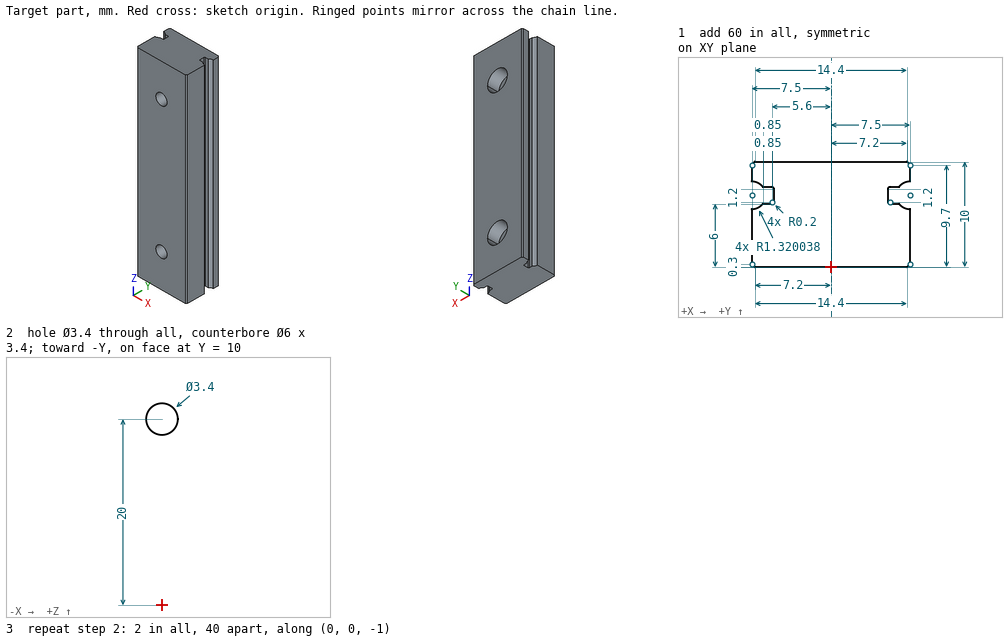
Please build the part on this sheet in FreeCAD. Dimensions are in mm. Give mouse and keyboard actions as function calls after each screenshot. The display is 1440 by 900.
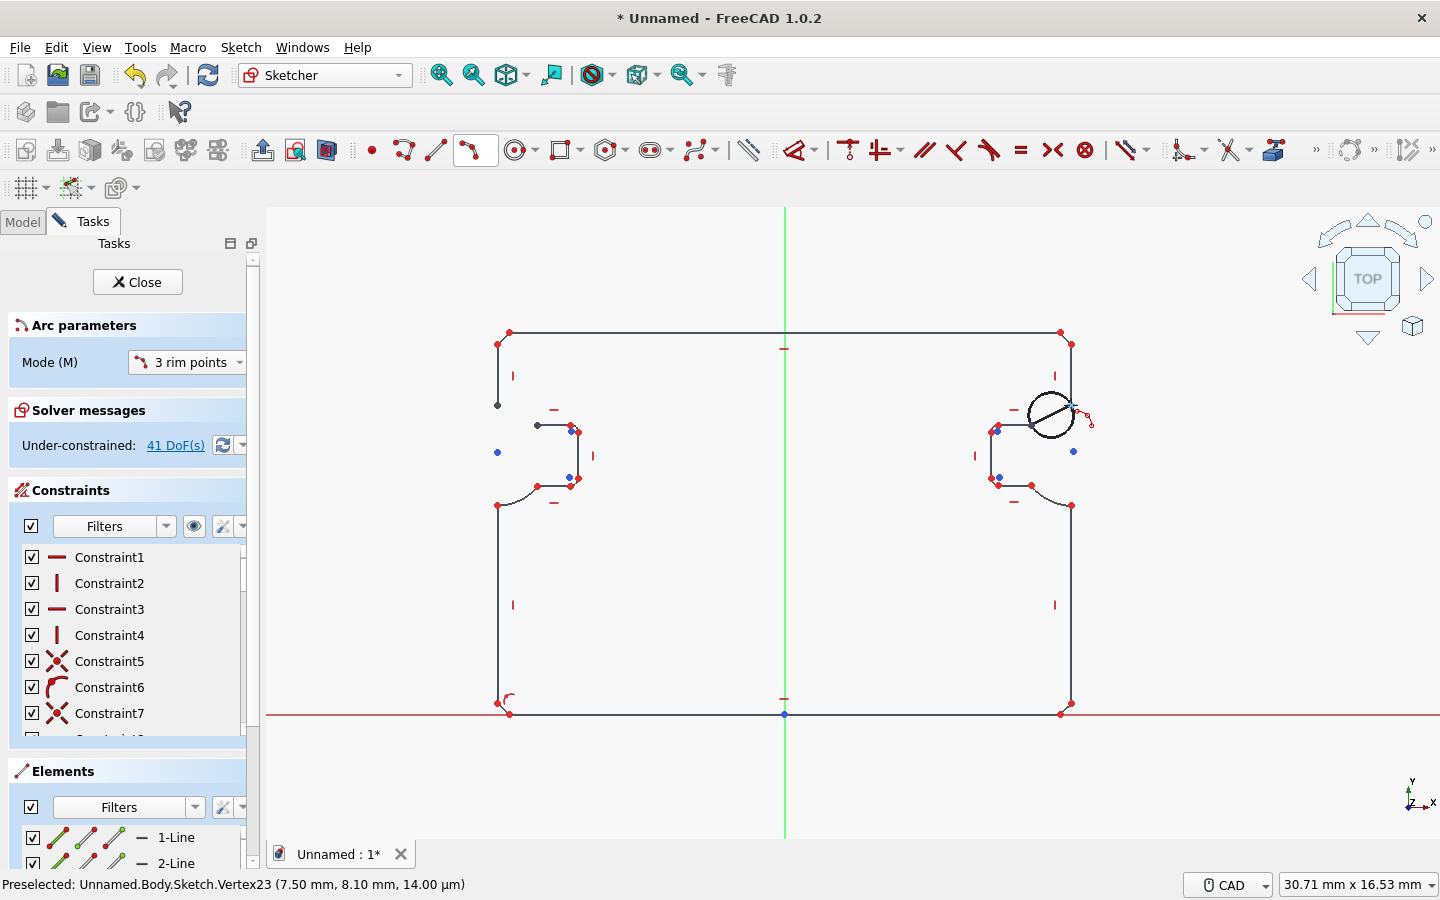
scroll(1049, 410, up, 6)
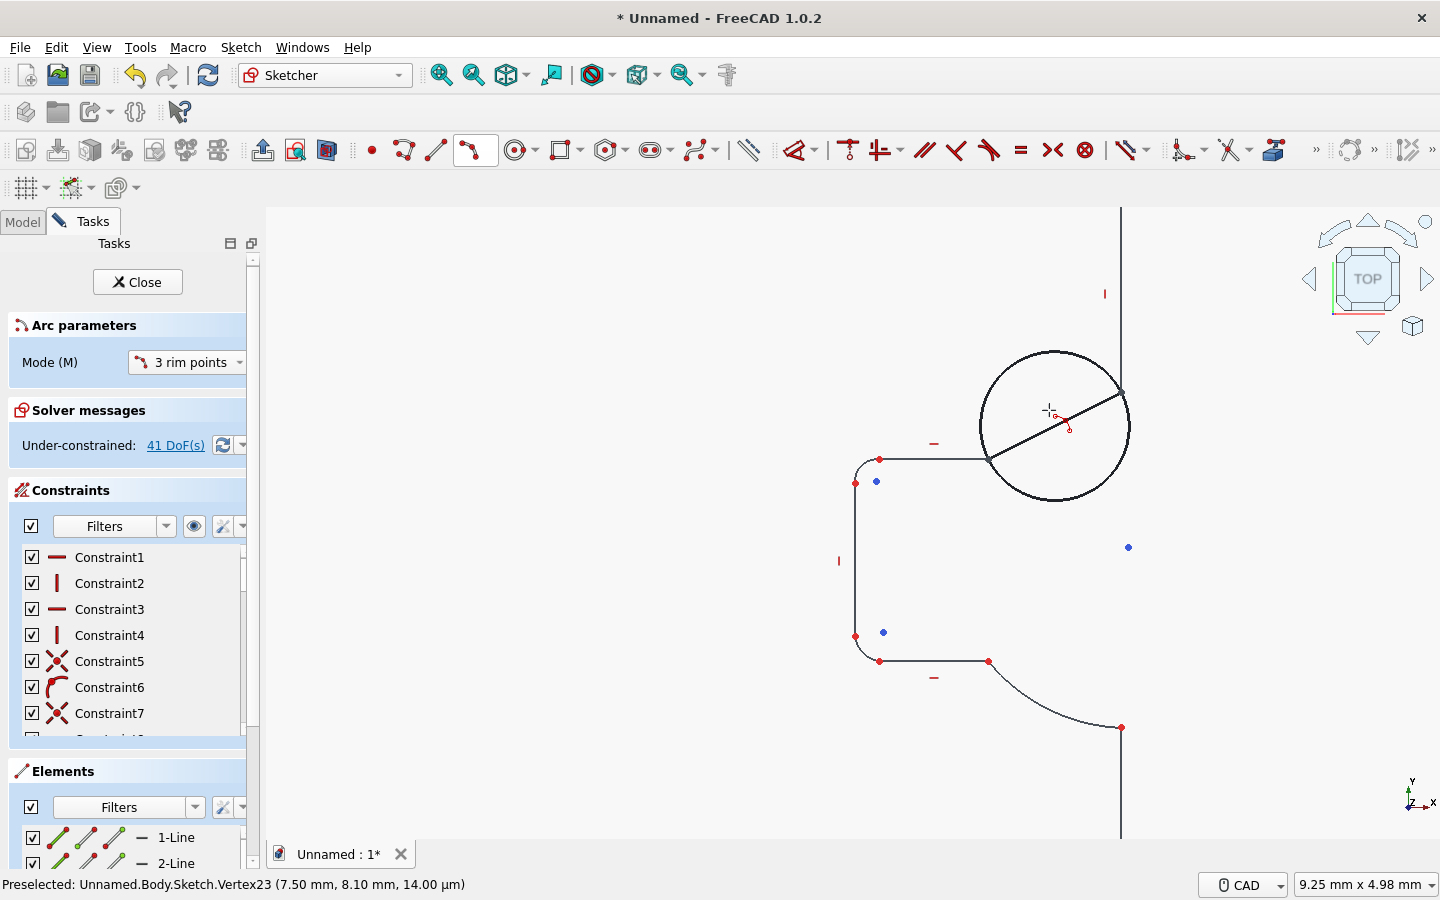
click(1047, 408)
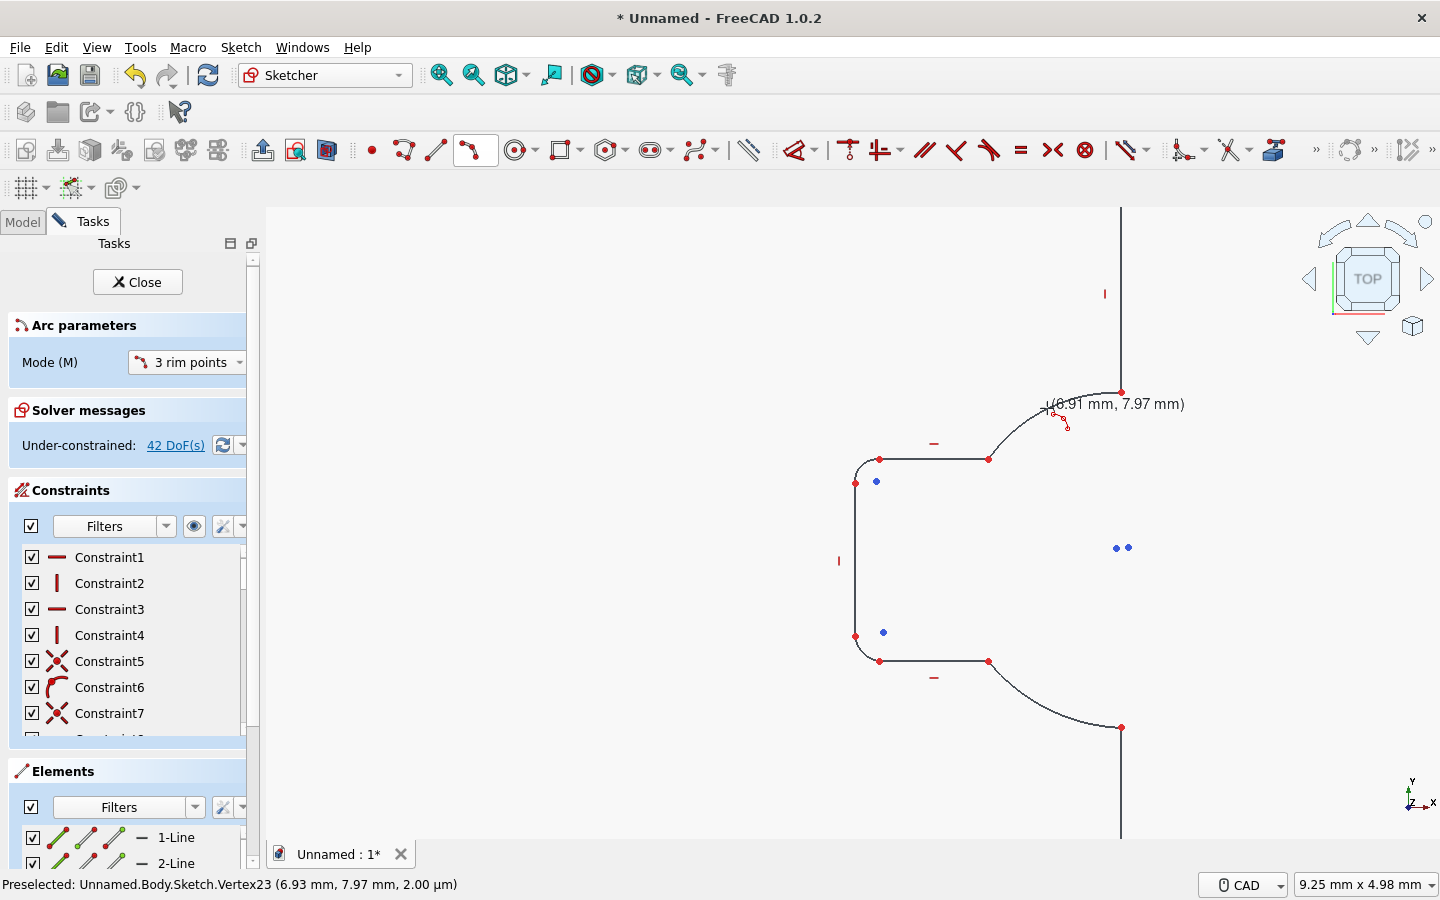
scroll(1049, 409, down, 6)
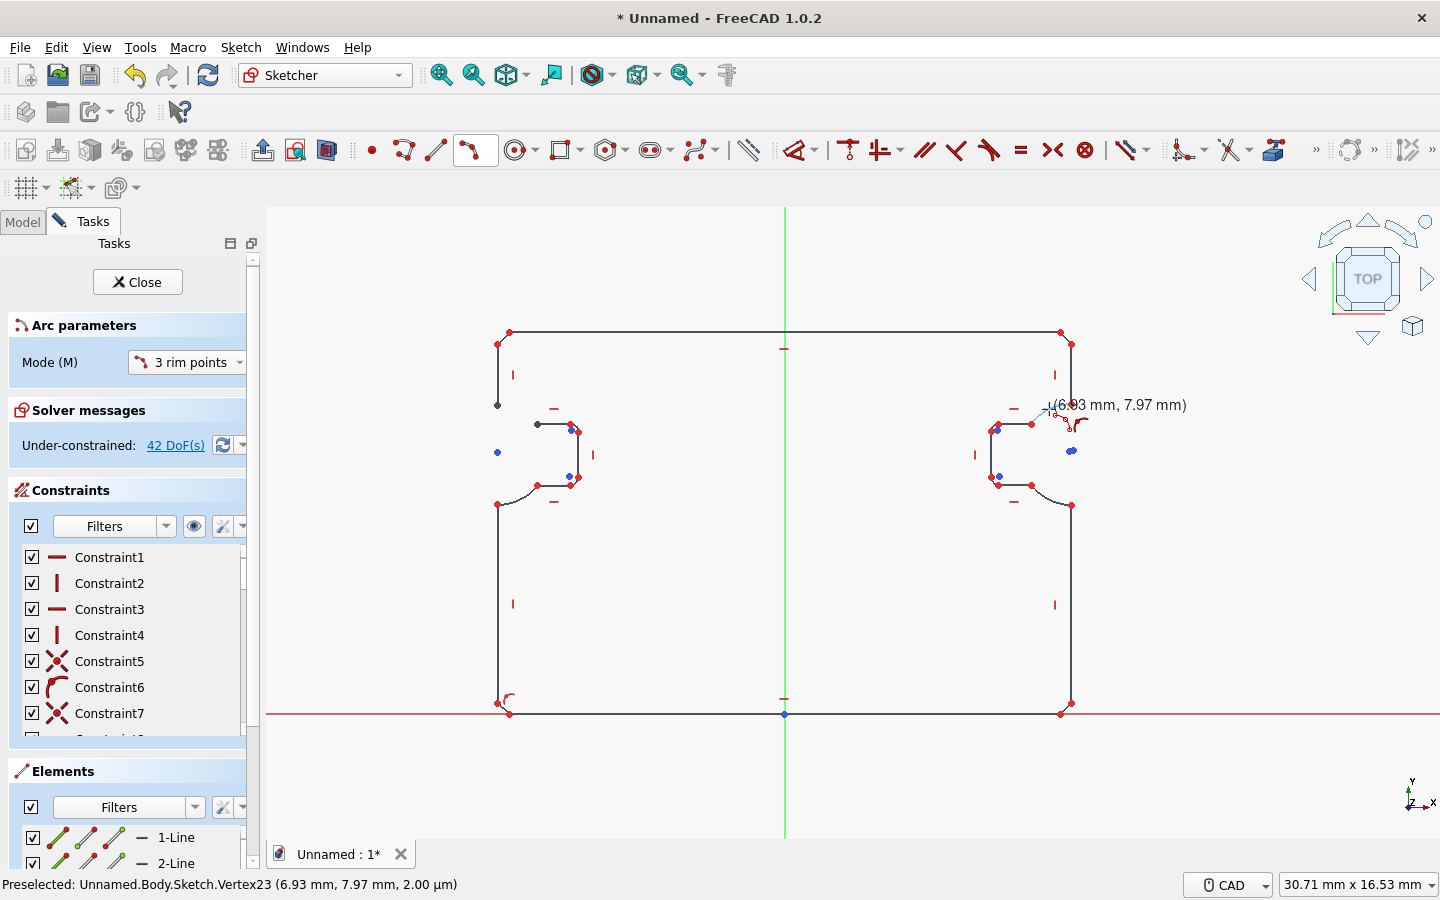
click(498, 405)
click(538, 424)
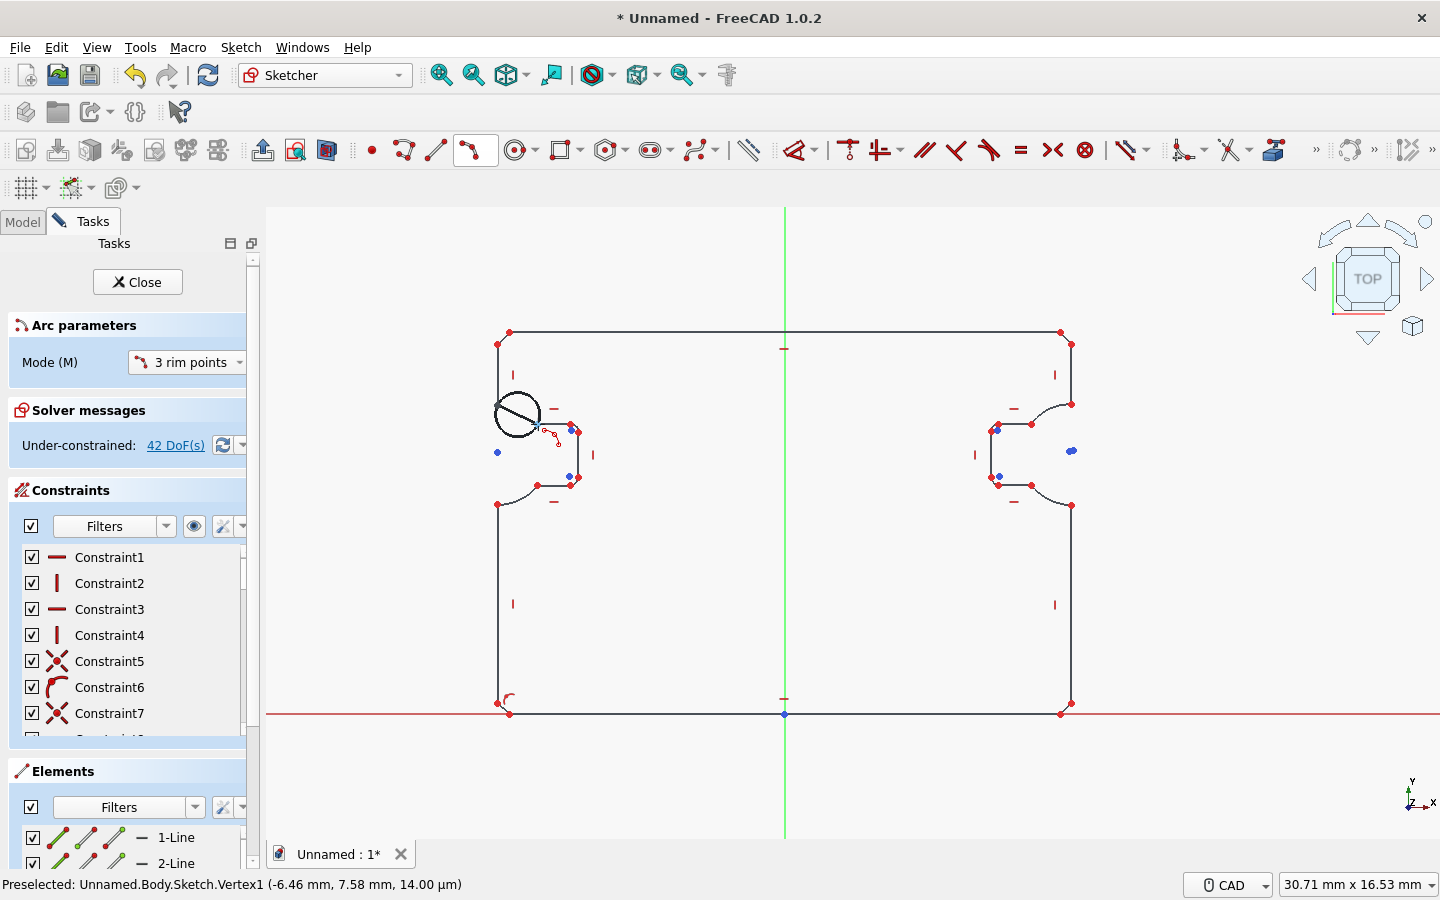
scroll(520, 409, up, 6)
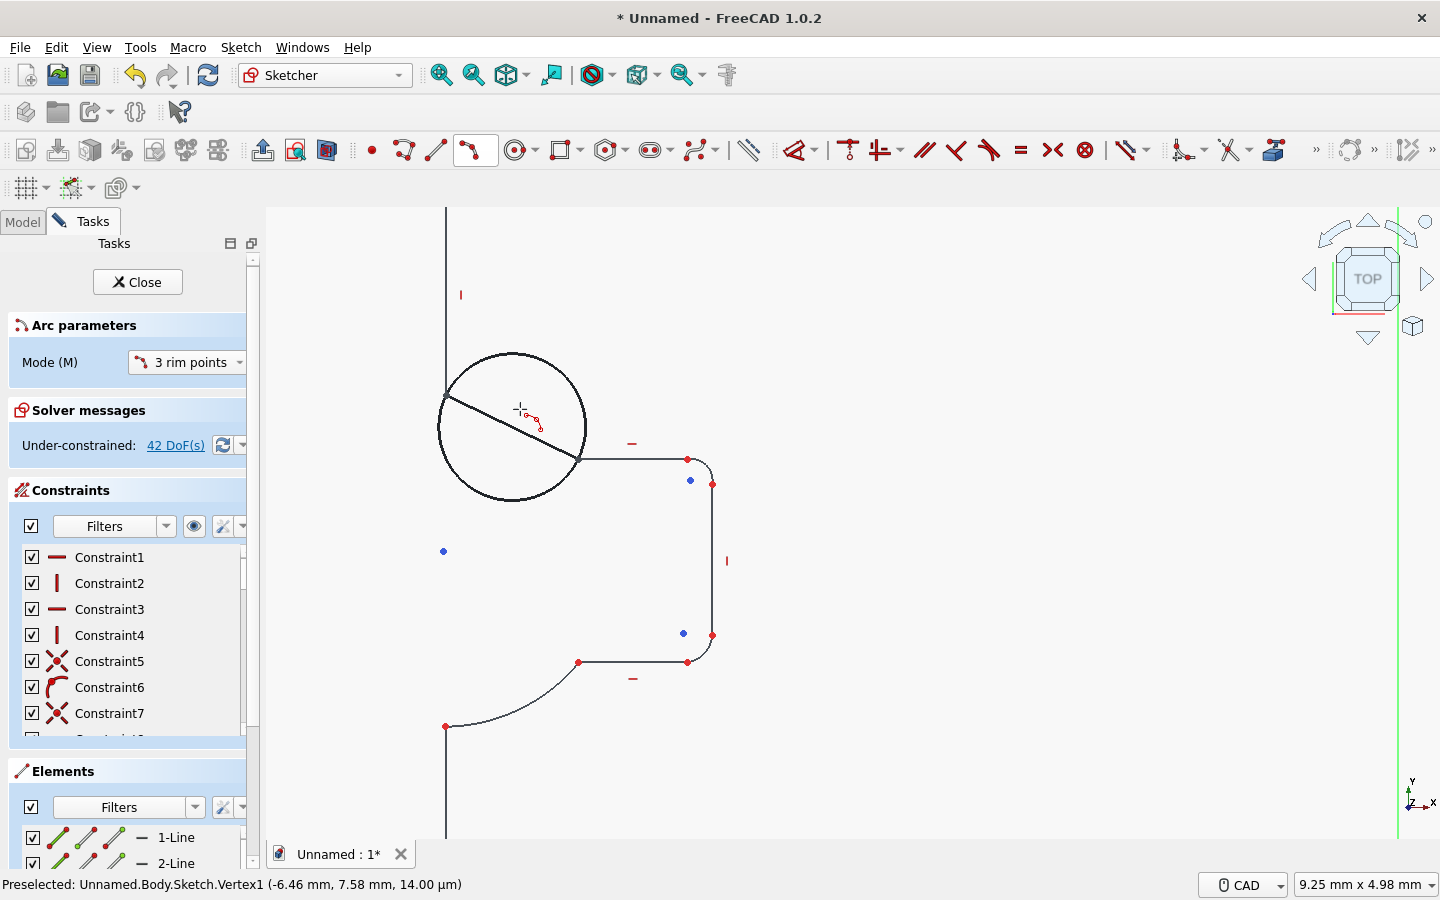
click(520, 408)
key(Escape)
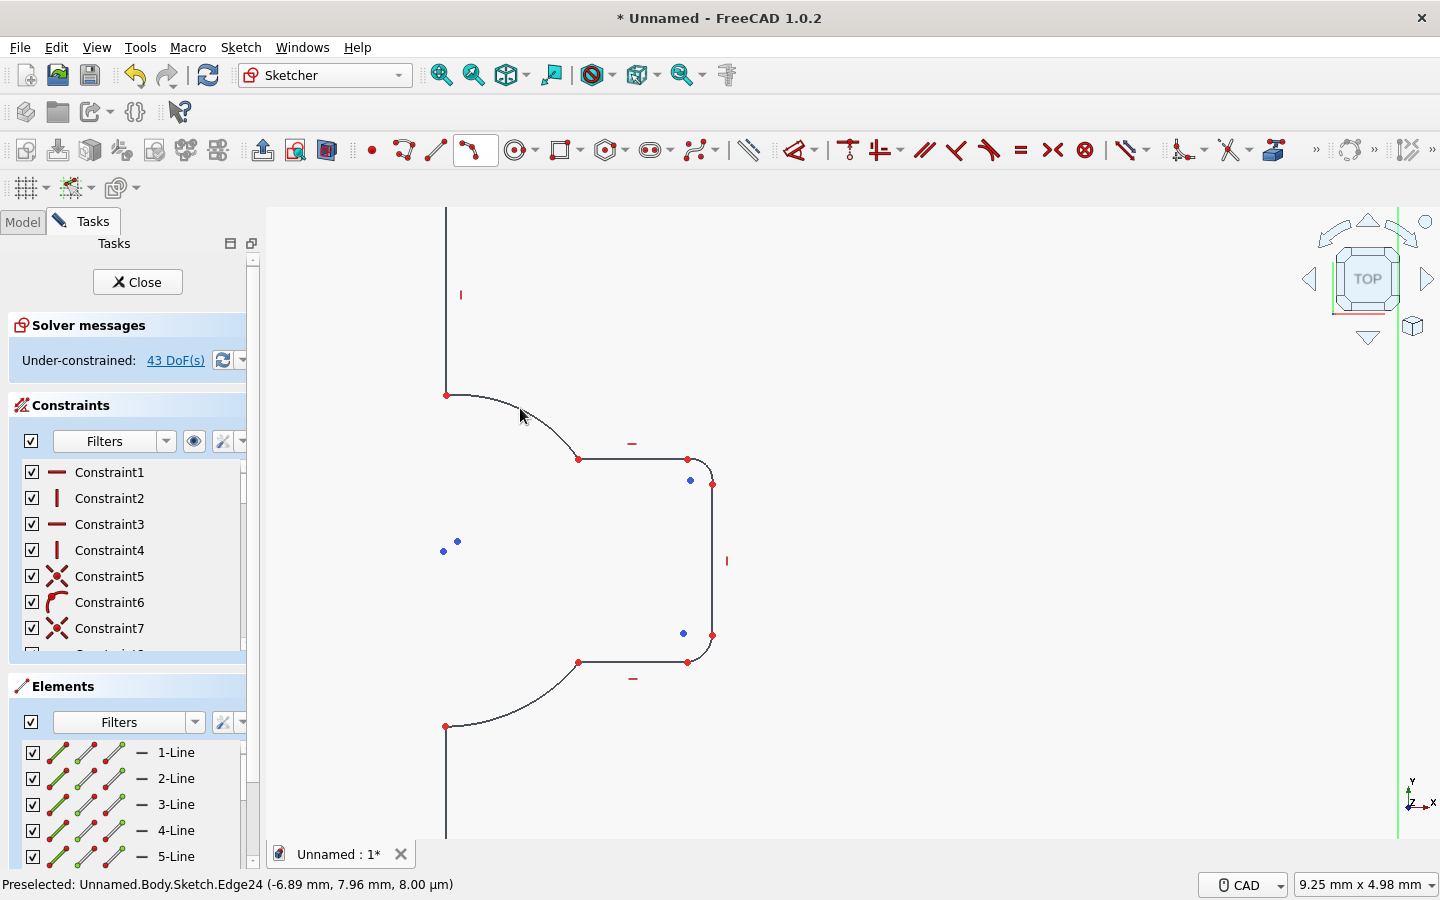
click(611, 459)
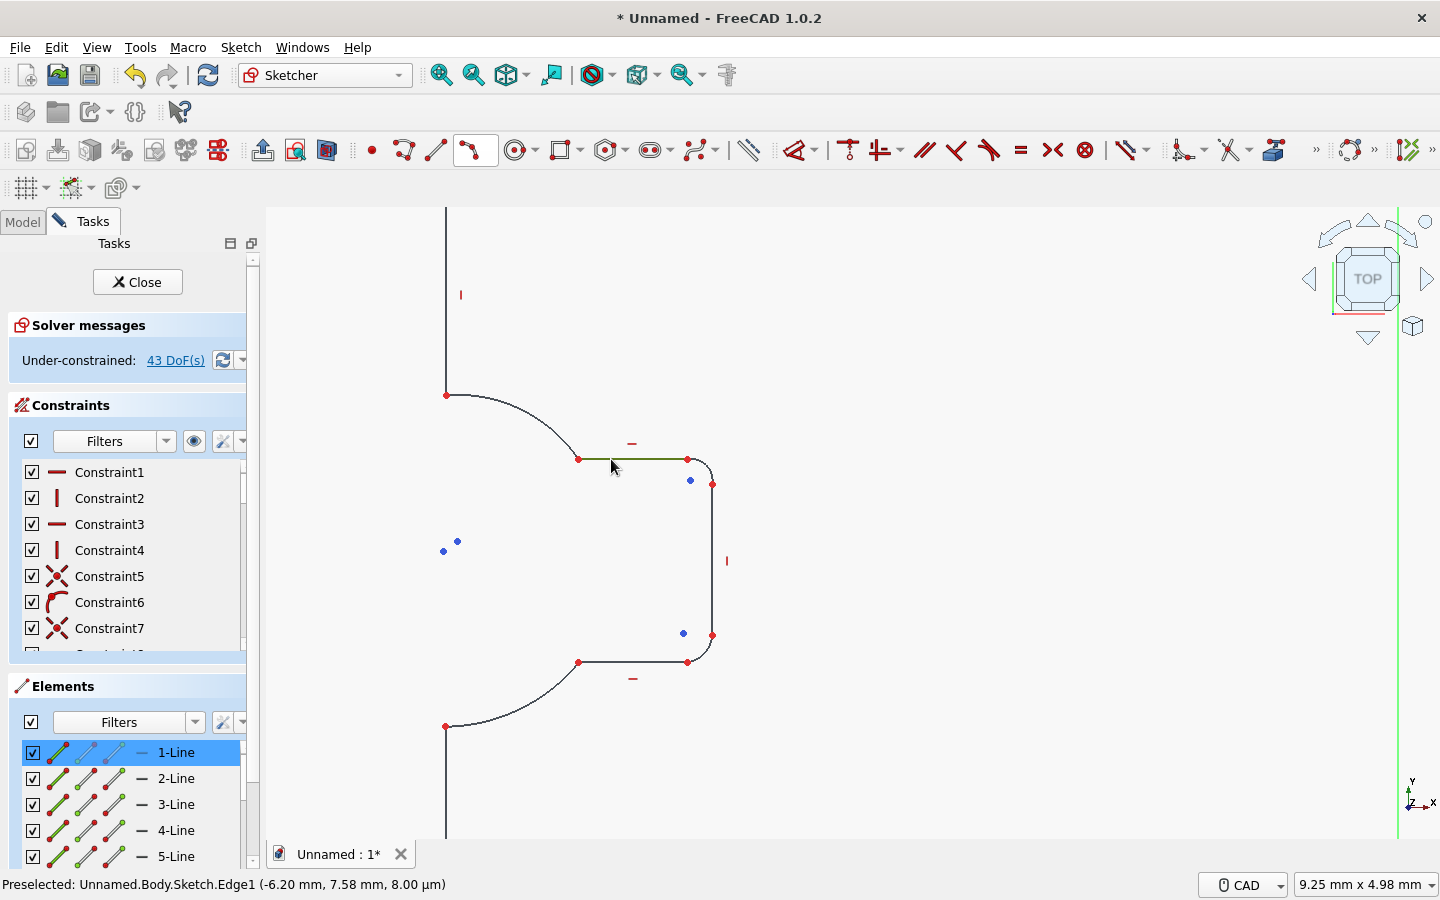
click(711, 473)